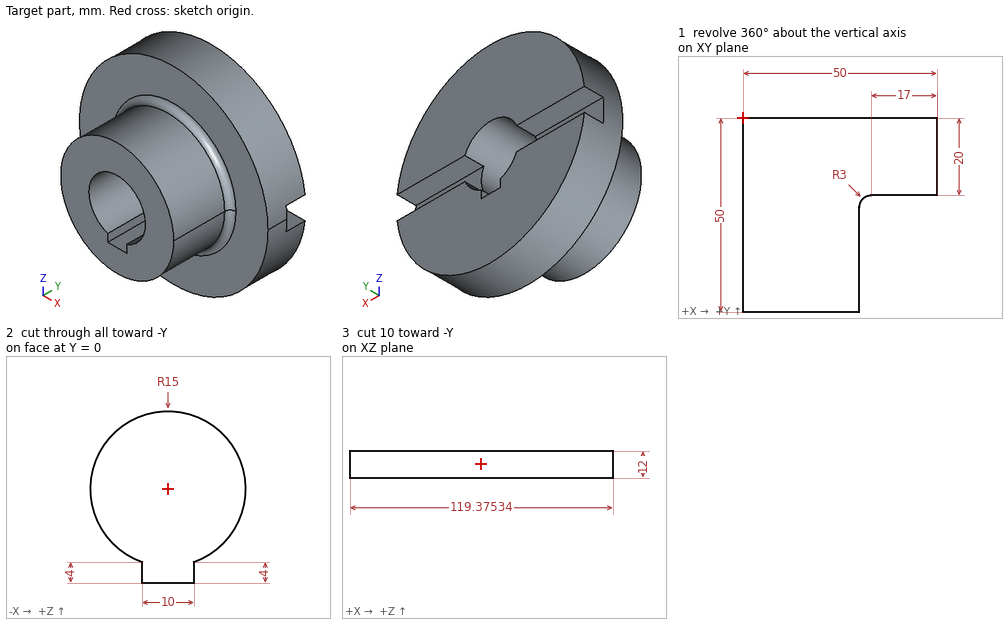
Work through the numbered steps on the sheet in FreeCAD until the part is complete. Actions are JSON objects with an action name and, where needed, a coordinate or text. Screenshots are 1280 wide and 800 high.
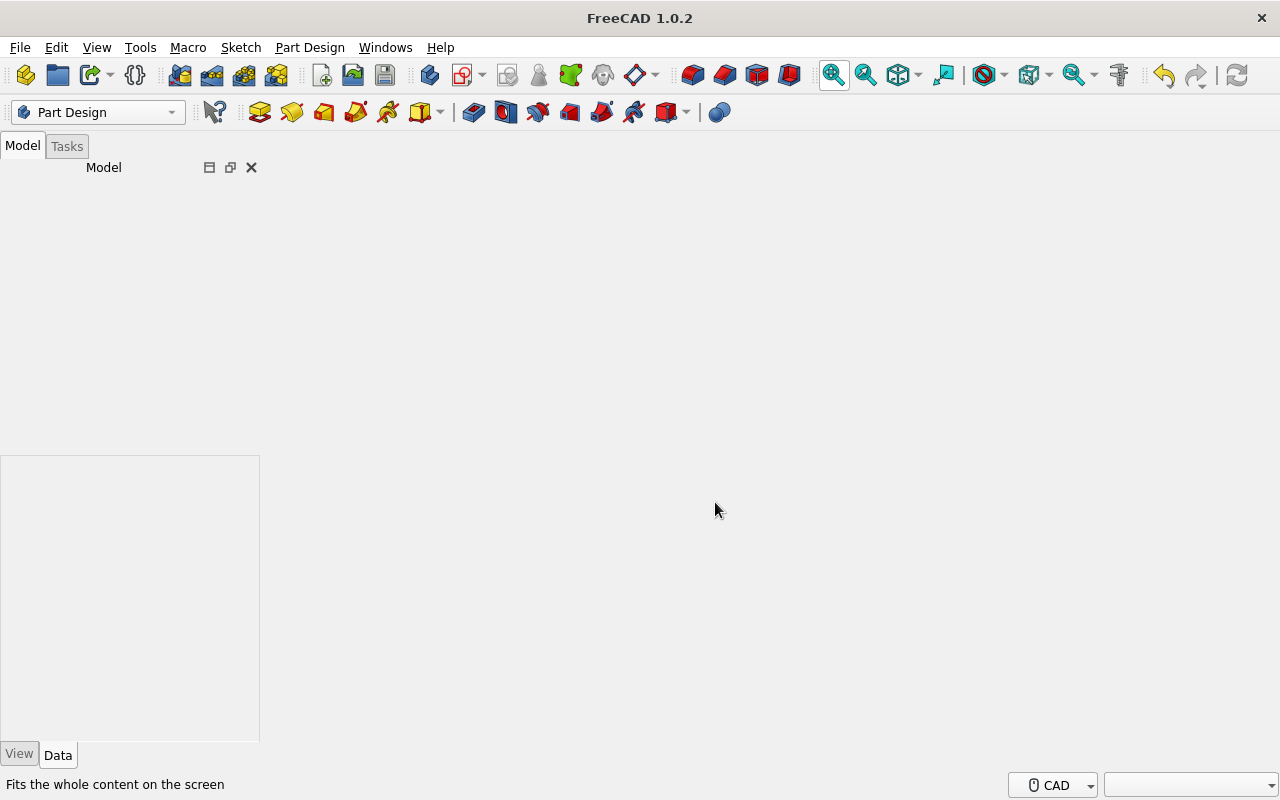
{"action": "left_click", "coordinate": [322, 76]}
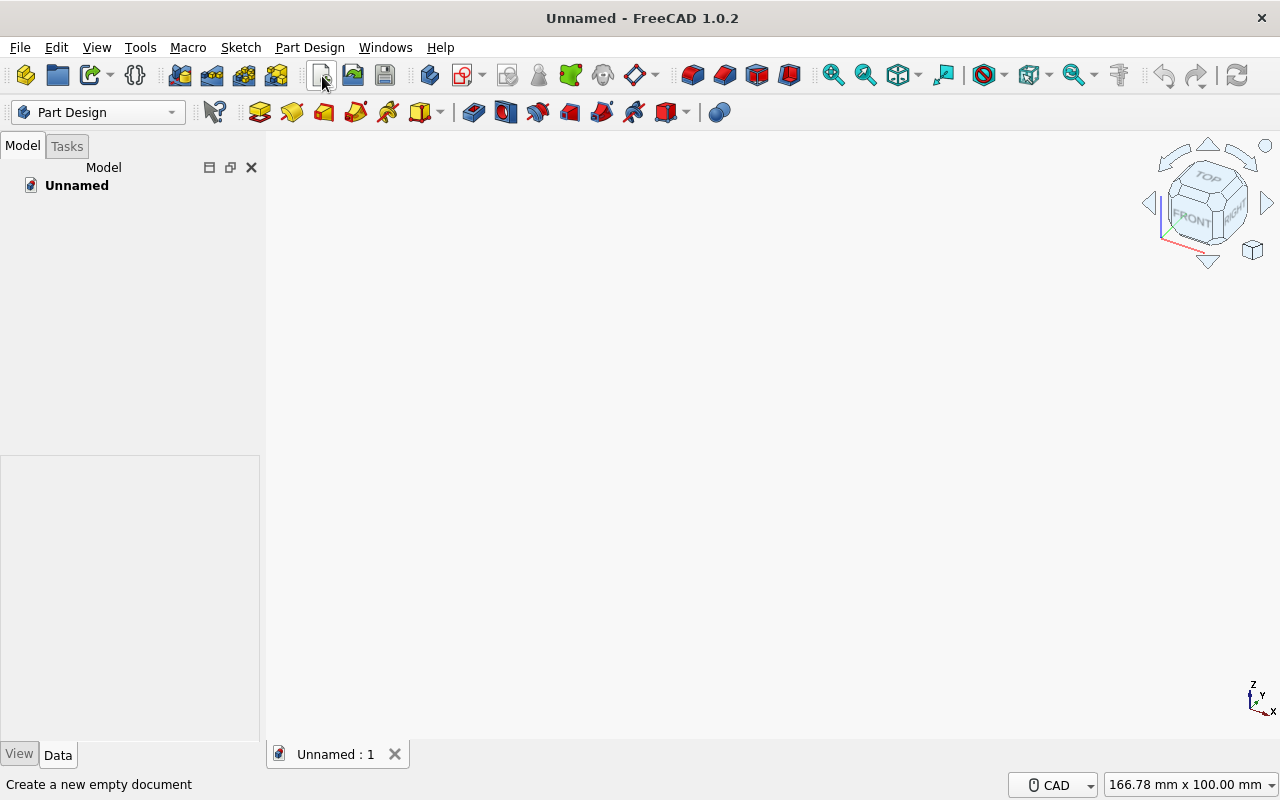
{"action": "left_click", "coordinate": [462, 76]}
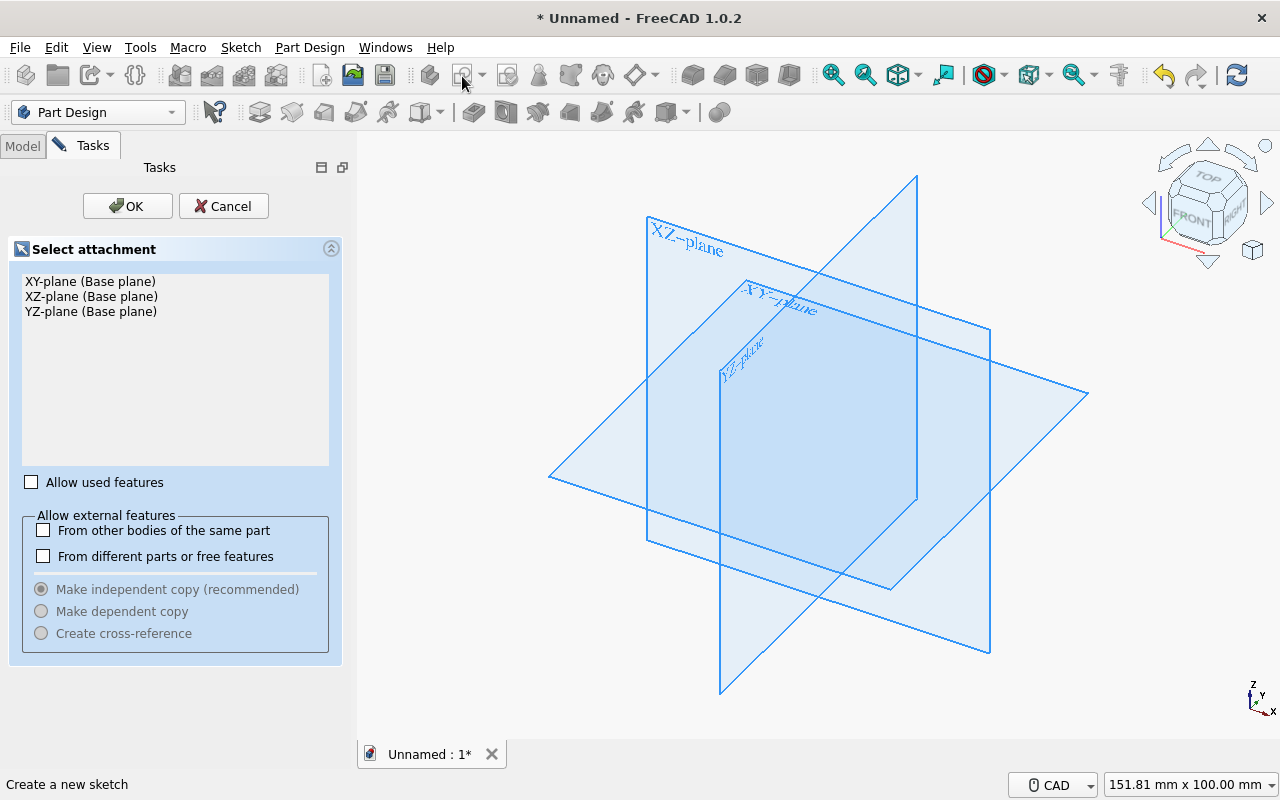
{"action": "left_click", "coordinate": [82, 282]}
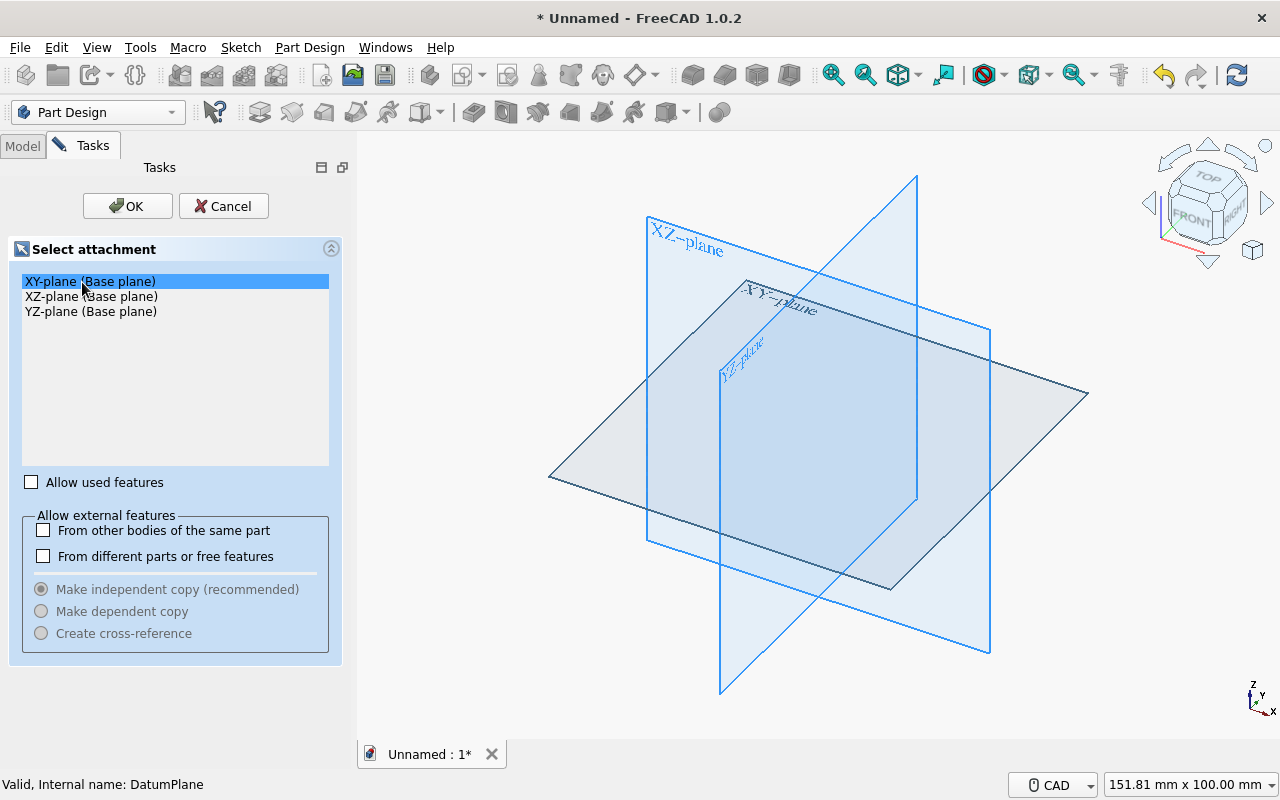
{"action": "left_click", "coordinate": [128, 206]}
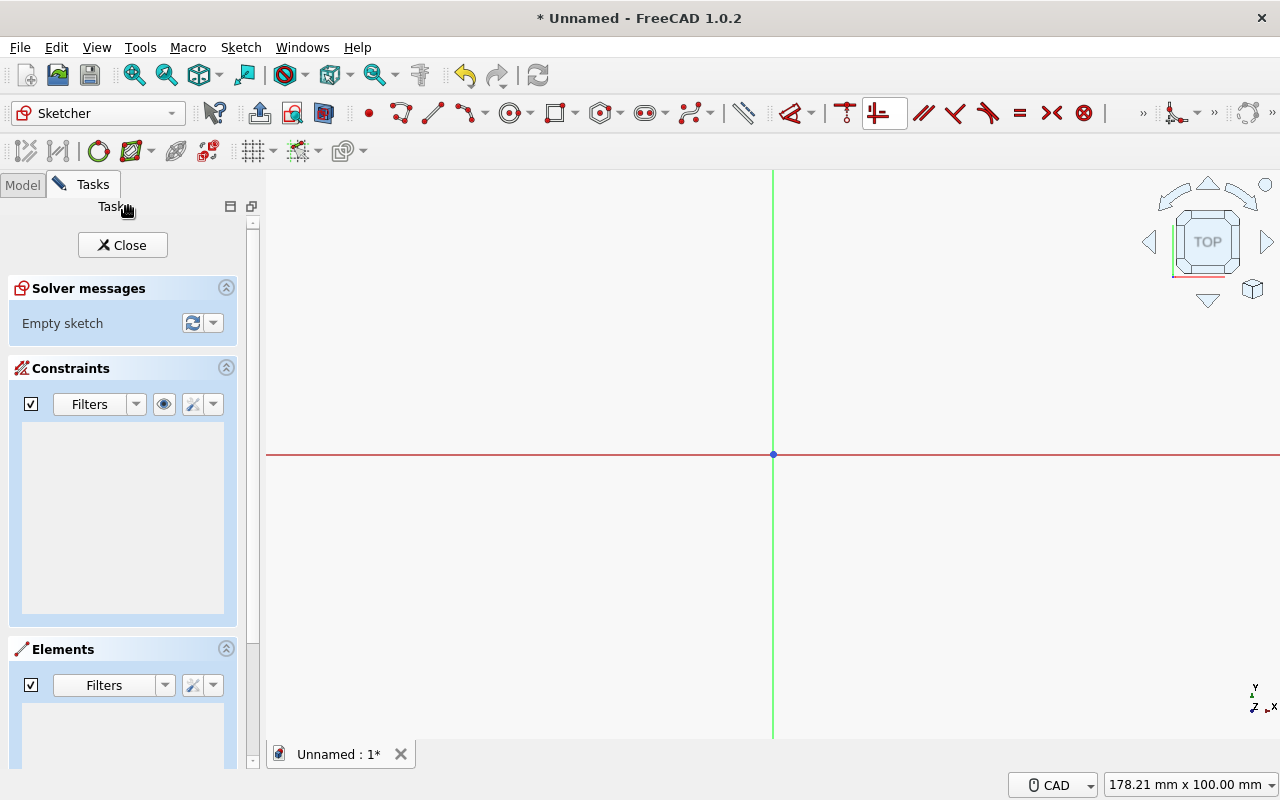
{"action": "scroll", "coordinate": [294, 198], "scroll_direction": "down", "scroll_amount": 1}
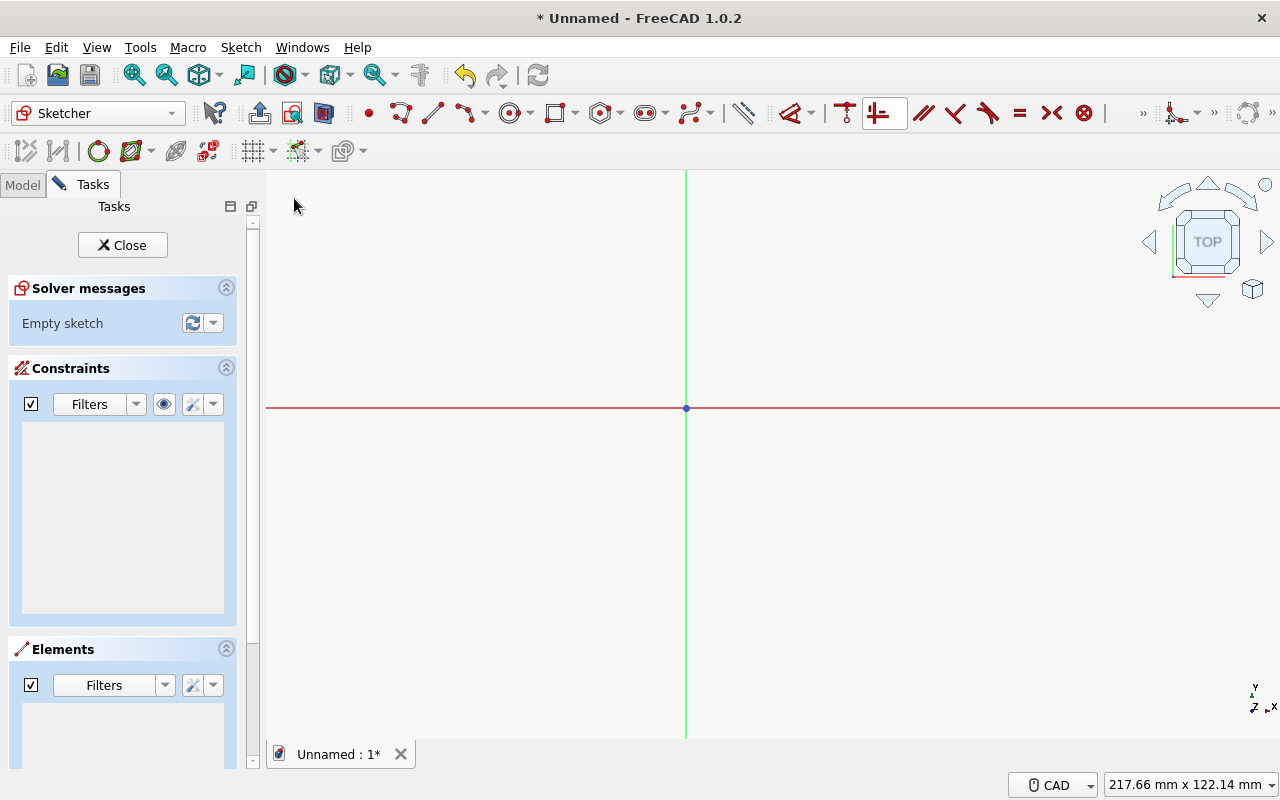
{"action": "scroll", "coordinate": [1002, 667], "scroll_direction": "up", "scroll_amount": 2}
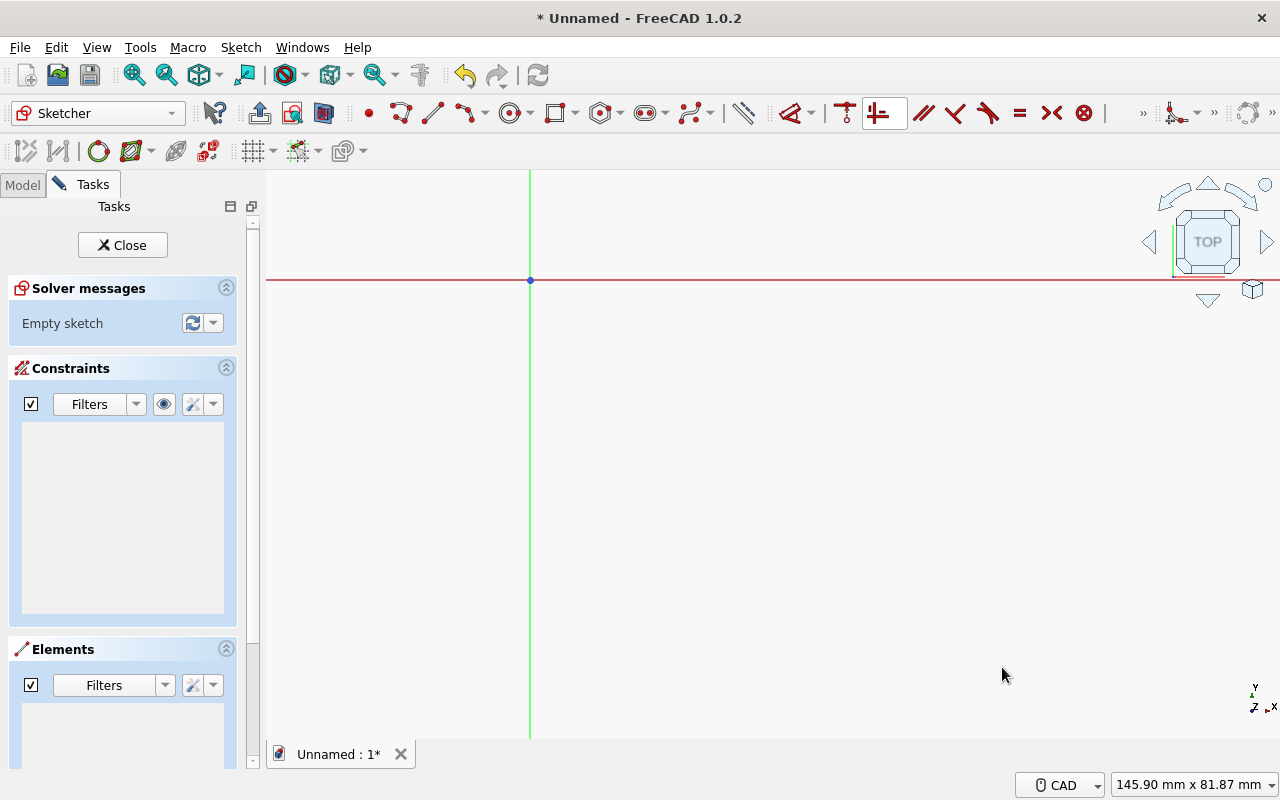
{"action": "left_click", "coordinate": [402, 114]}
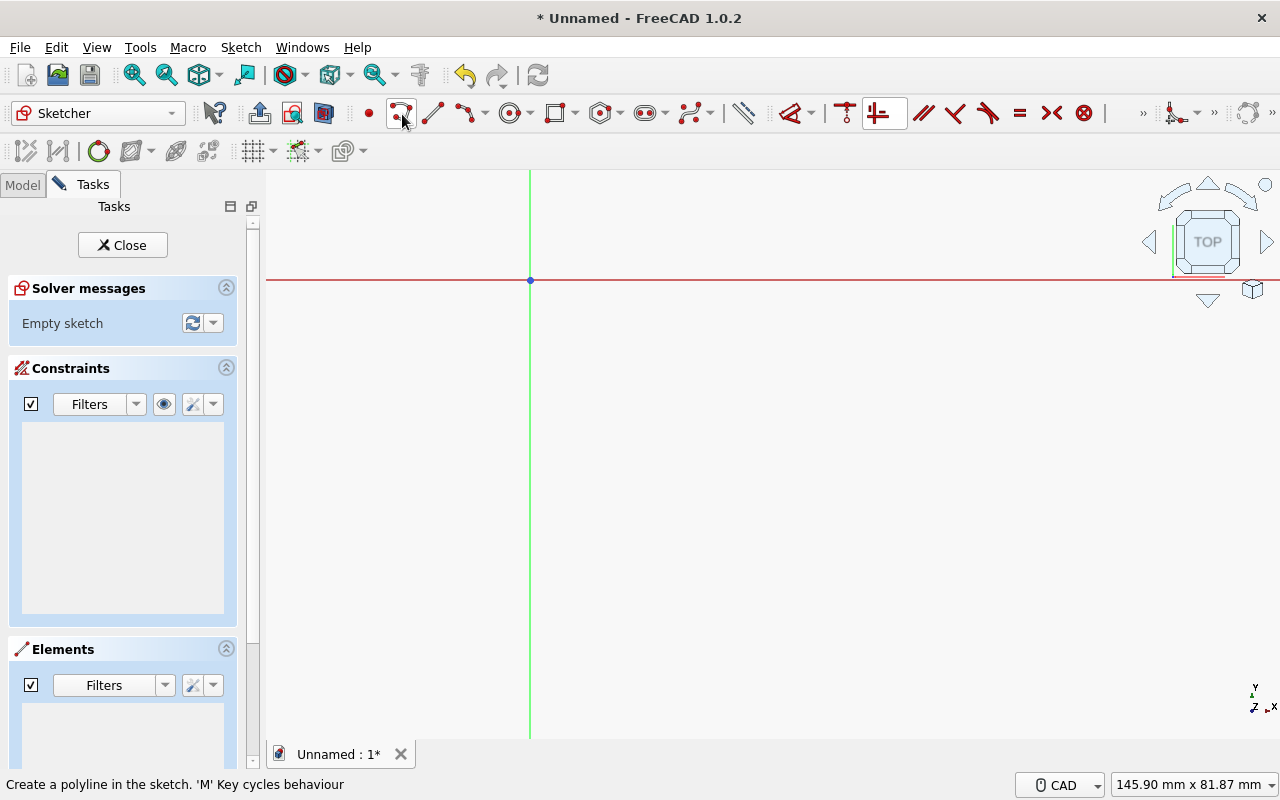
{"action": "left_click", "coordinate": [760, 419]}
{"action": "left_click", "coordinate": [878, 419]}
{"action": "left_click", "coordinate": [878, 280]}
{"action": "left_click", "coordinate": [530, 280]}
{"action": "left_click", "coordinate": [539, 628]}
{"action": "left_click", "coordinate": [739, 628]}
{"action": "left_click", "coordinate": [739, 440]}
{"action": "right_click", "coordinate": [739, 440]}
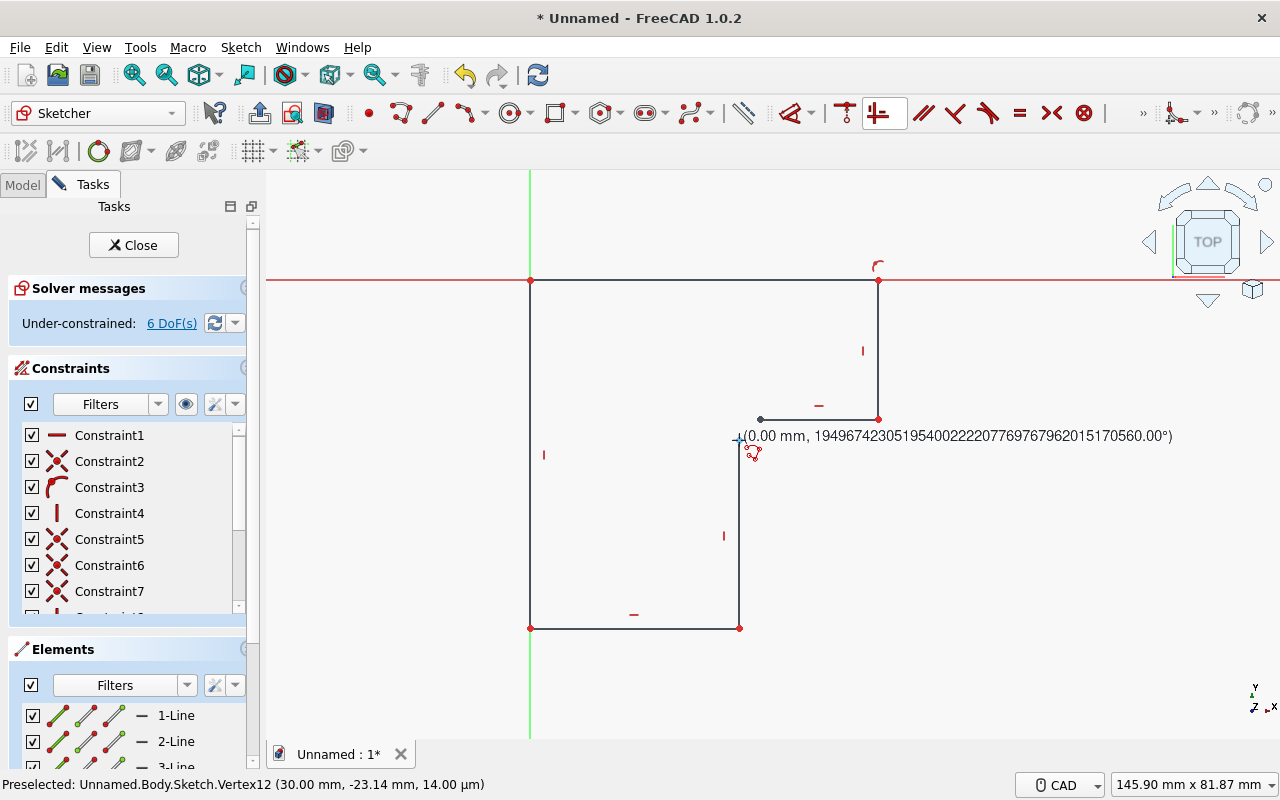
{"action": "left_click", "coordinate": [466, 114]}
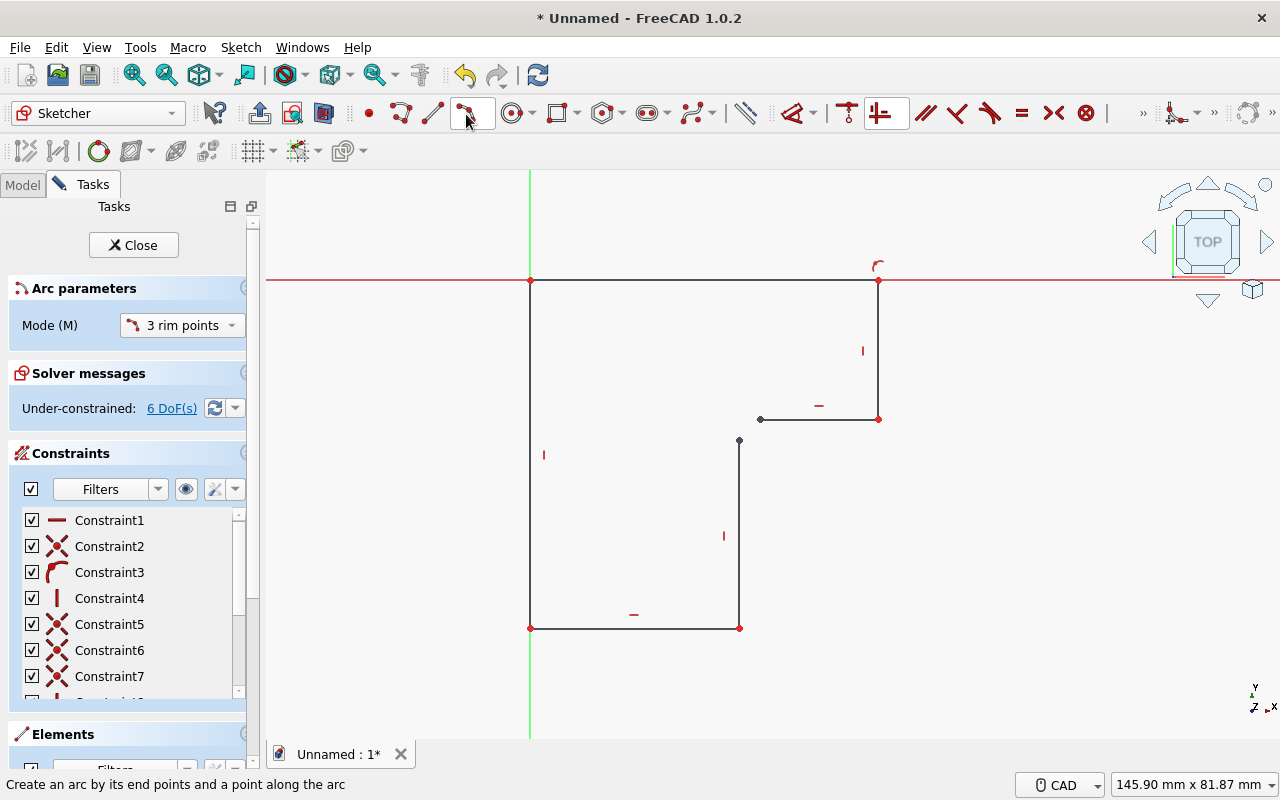
{"action": "left_click", "coordinate": [739, 441]}
{"action": "left_click", "coordinate": [760, 420]}